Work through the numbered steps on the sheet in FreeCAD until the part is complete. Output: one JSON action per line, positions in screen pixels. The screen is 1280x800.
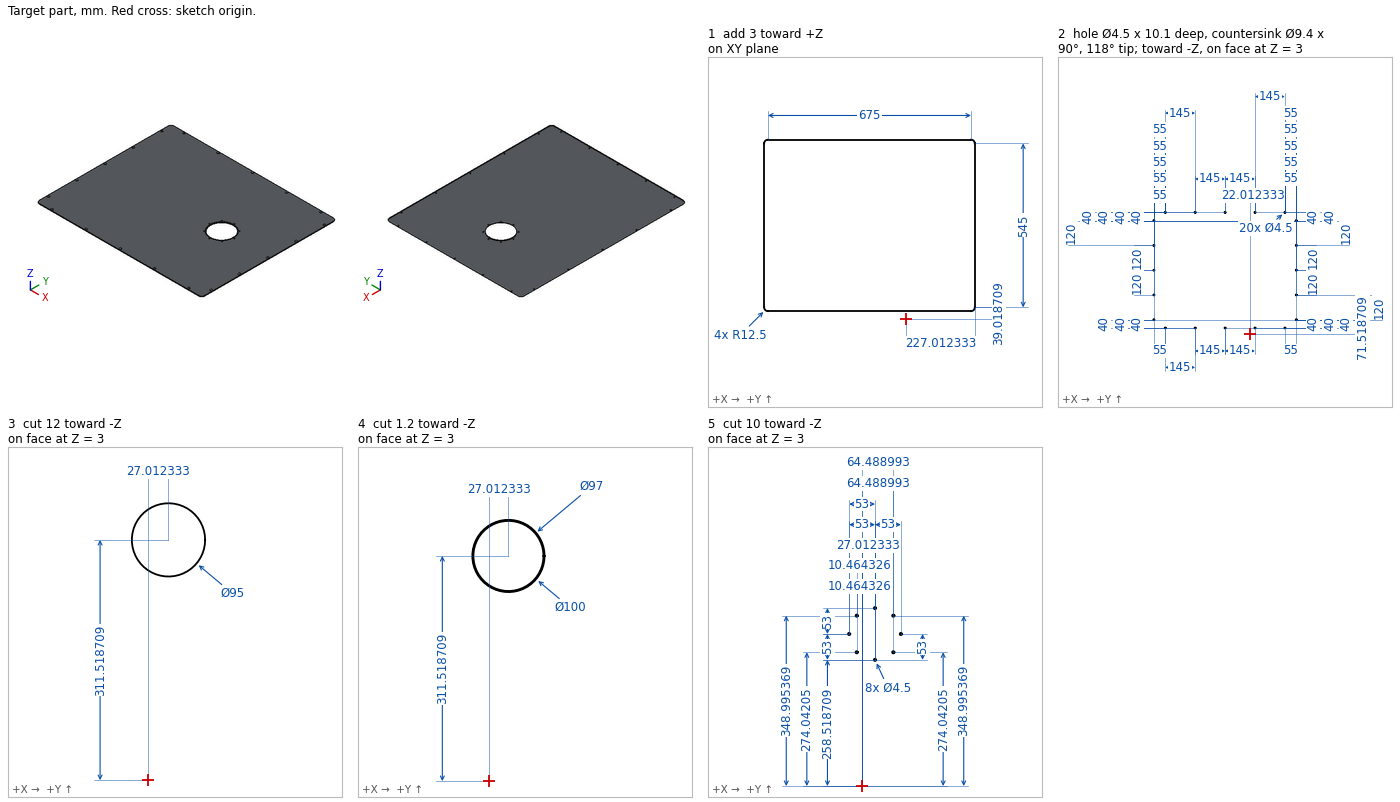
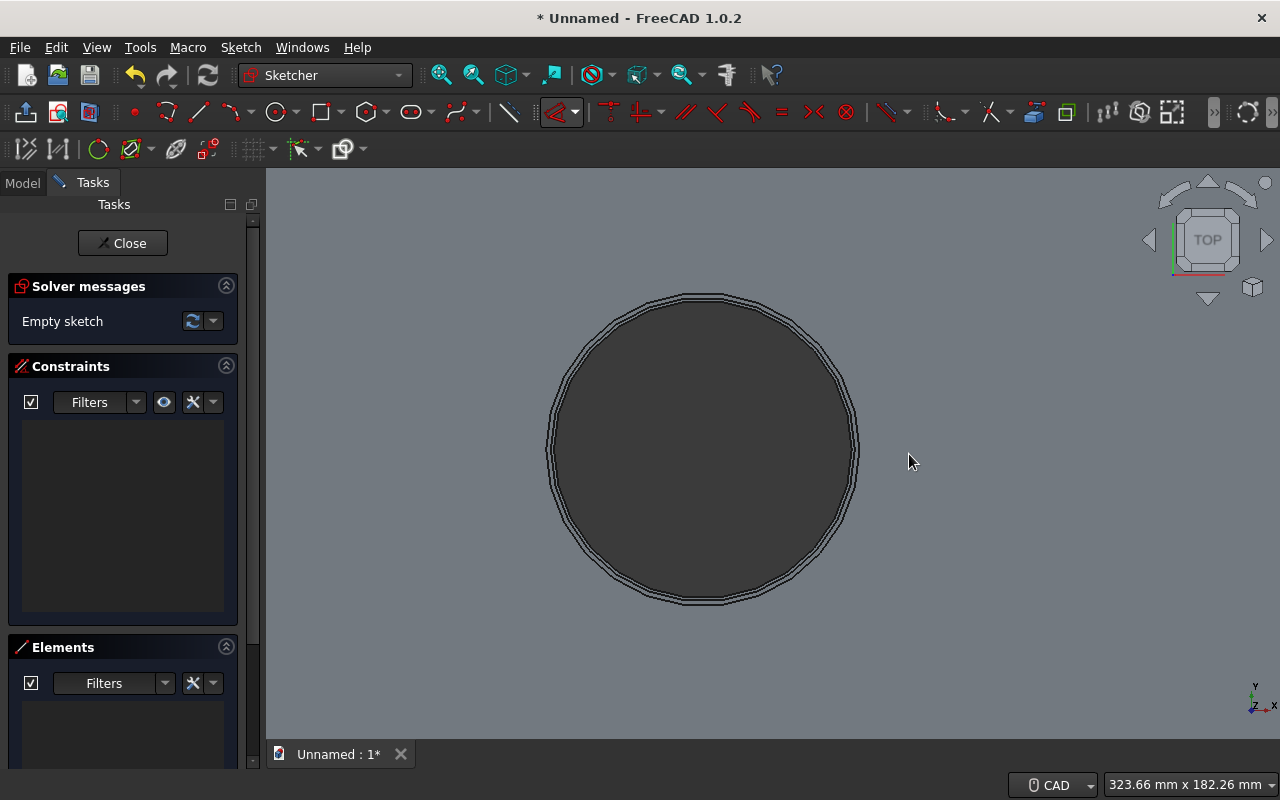
{"action": "left_click", "coordinate": [276, 112]}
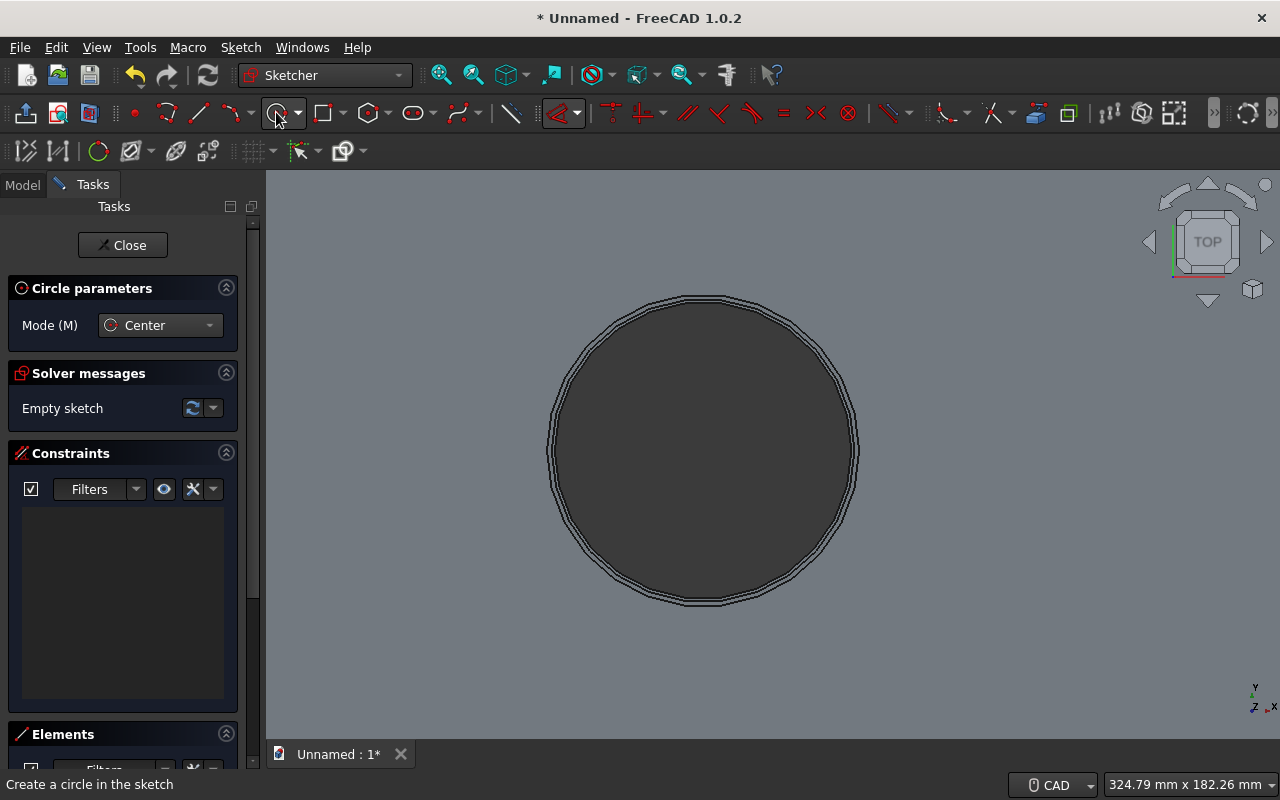
{"action": "scroll", "coordinate": [703, 616], "scroll_direction": "up", "scroll_amount": 6}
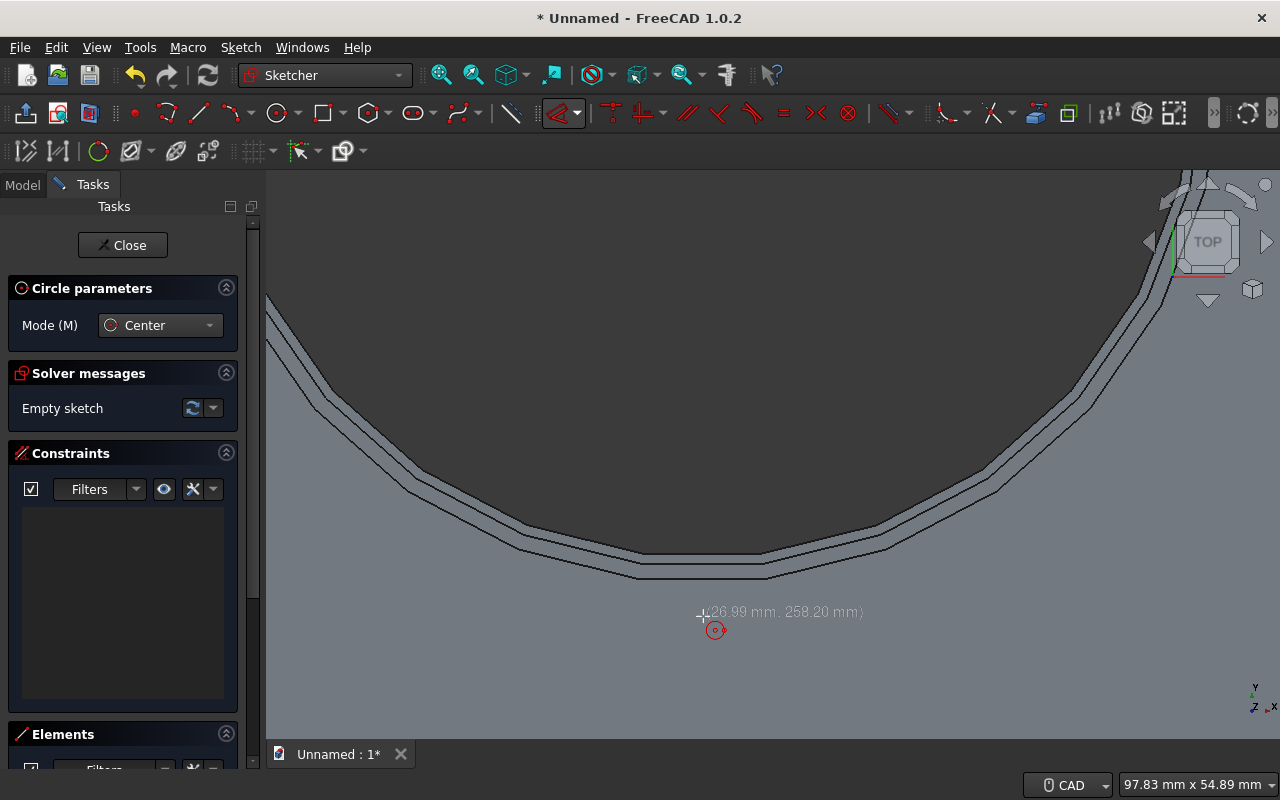
{"action": "left_click", "coordinate": [702, 614]}
{"action": "left_click", "coordinate": [719, 598]}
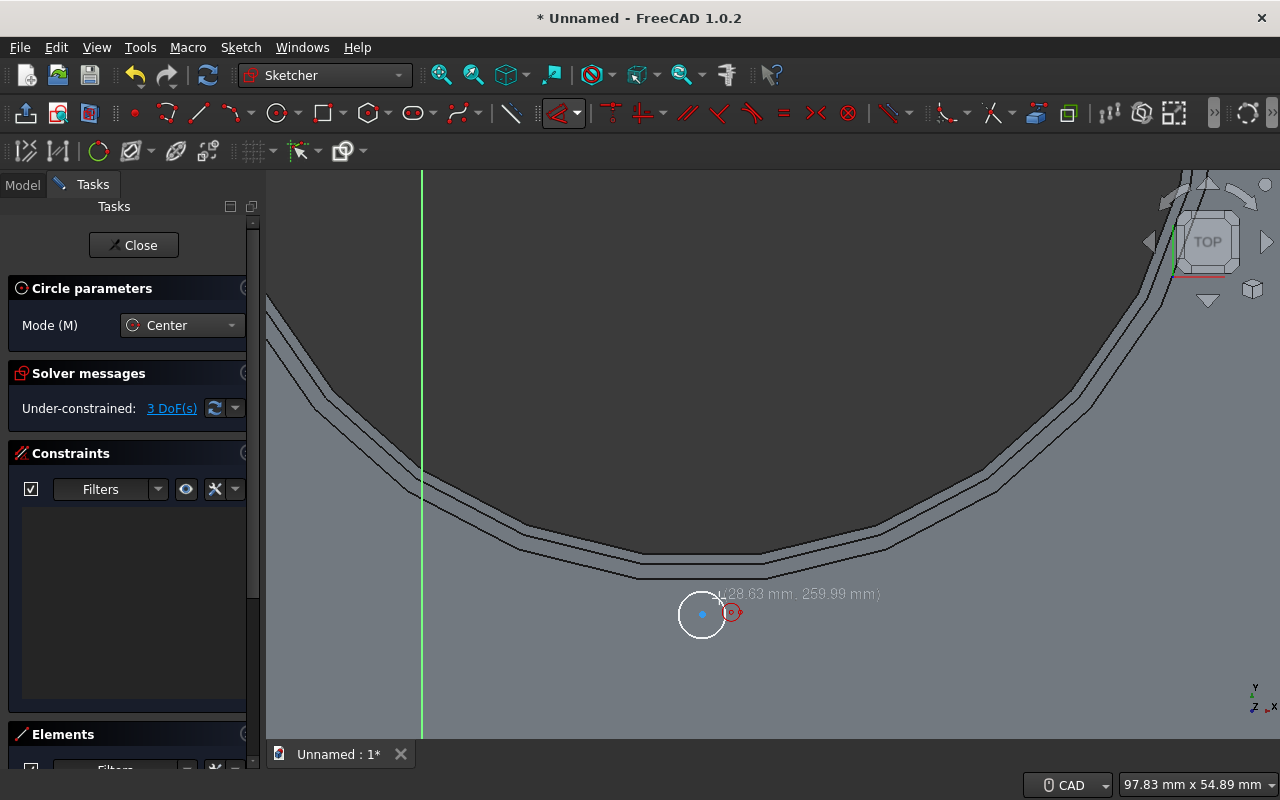
{"action": "left_click", "coordinate": [314, 453]}
{"action": "left_click", "coordinate": [330, 437]}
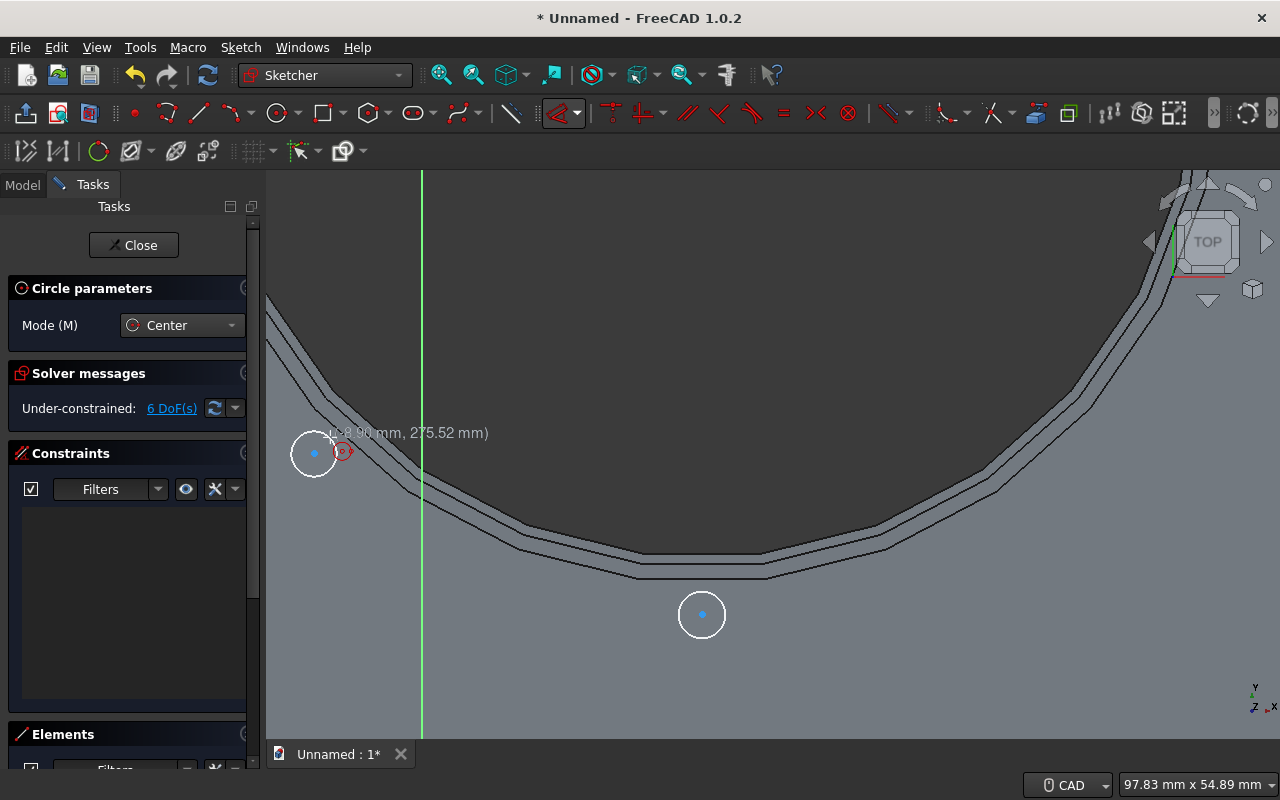
{"action": "scroll", "coordinate": [705, 622], "scroll_direction": "down", "scroll_amount": 6}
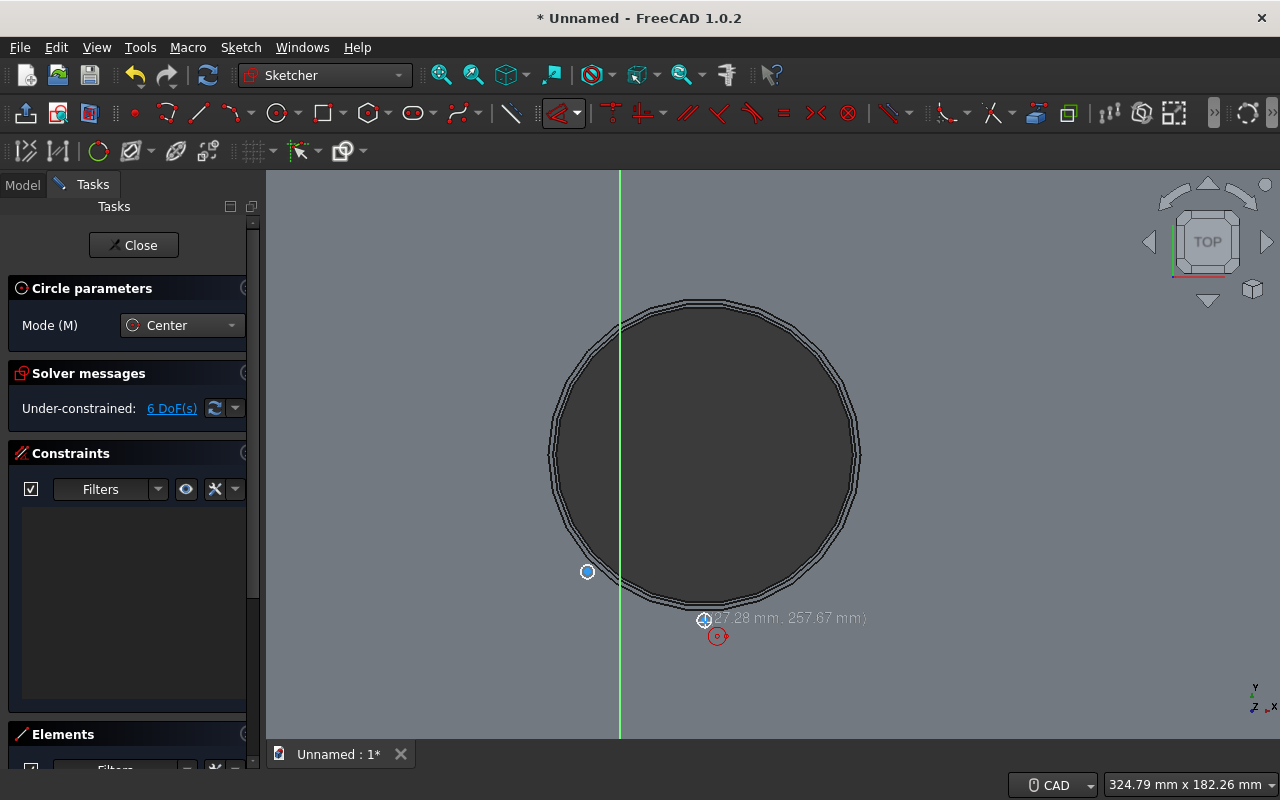
{"action": "scroll", "coordinate": [539, 455], "scroll_direction": "up", "scroll_amount": 6}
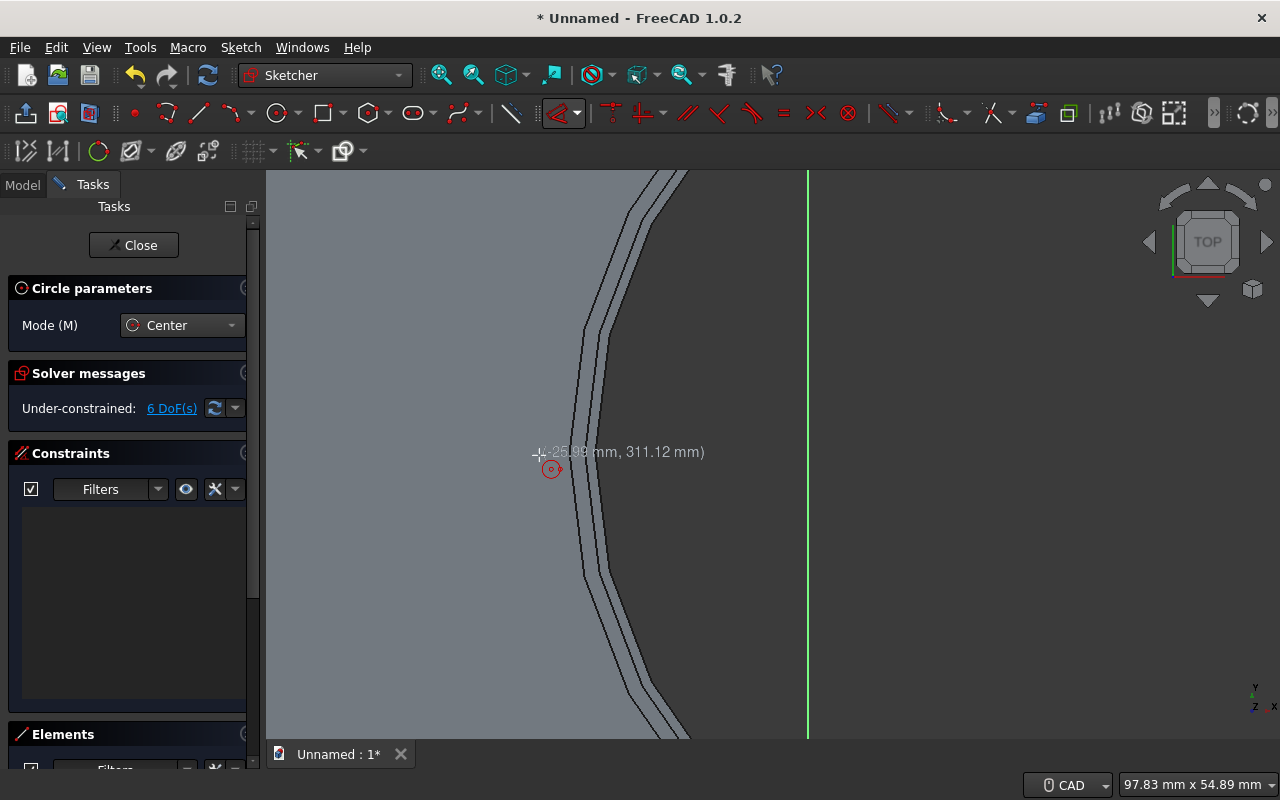
{"action": "left_click", "coordinate": [538, 453]}
{"action": "left_click", "coordinate": [555, 437]}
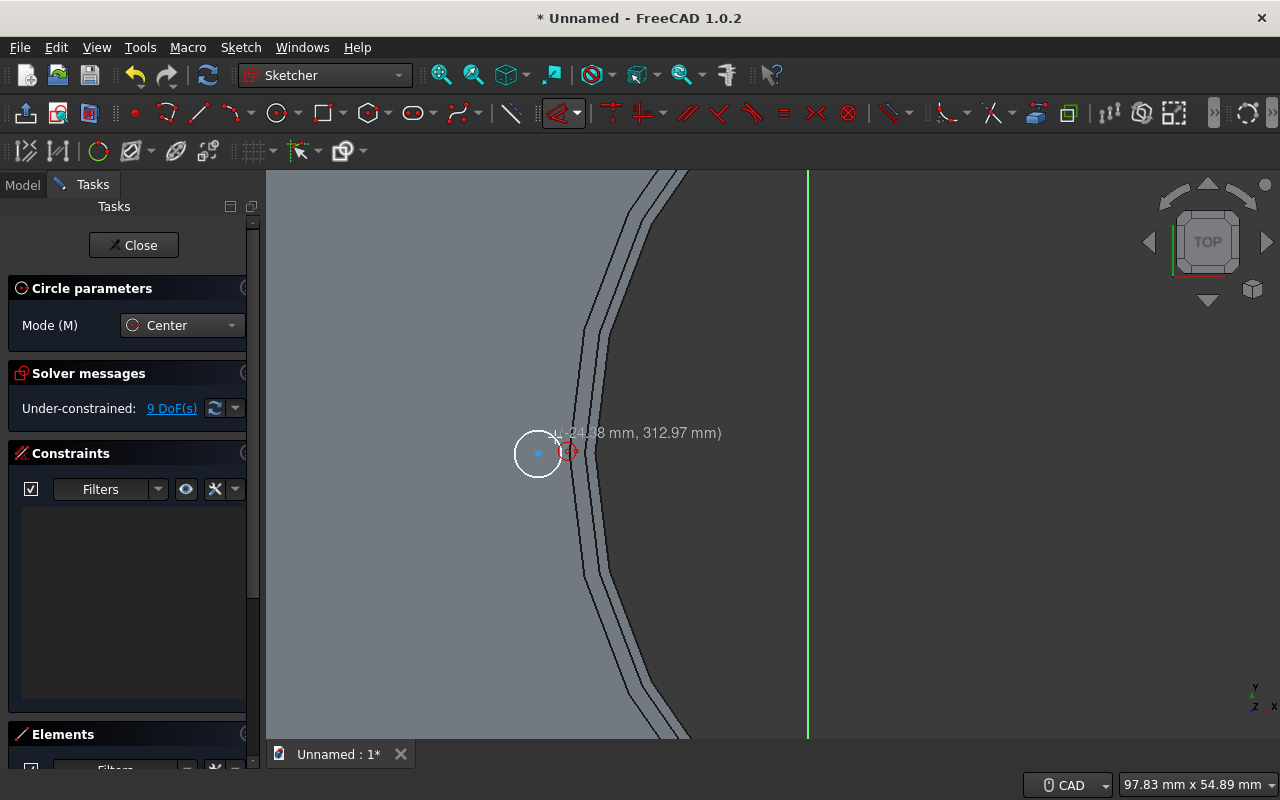
{"action": "scroll", "coordinate": [539, 455], "scroll_direction": "down", "scroll_amount": 6}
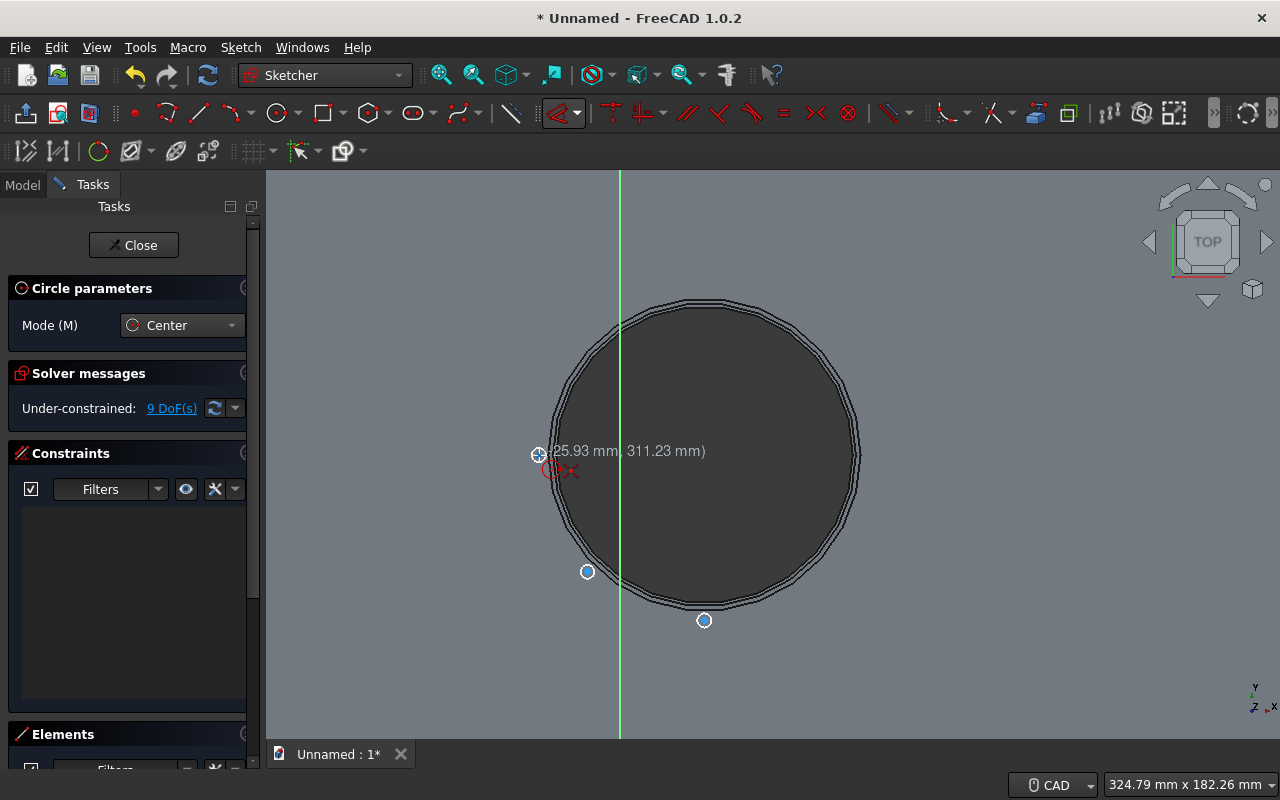
{"action": "scroll", "coordinate": [587, 338], "scroll_direction": "up", "scroll_amount": 6}